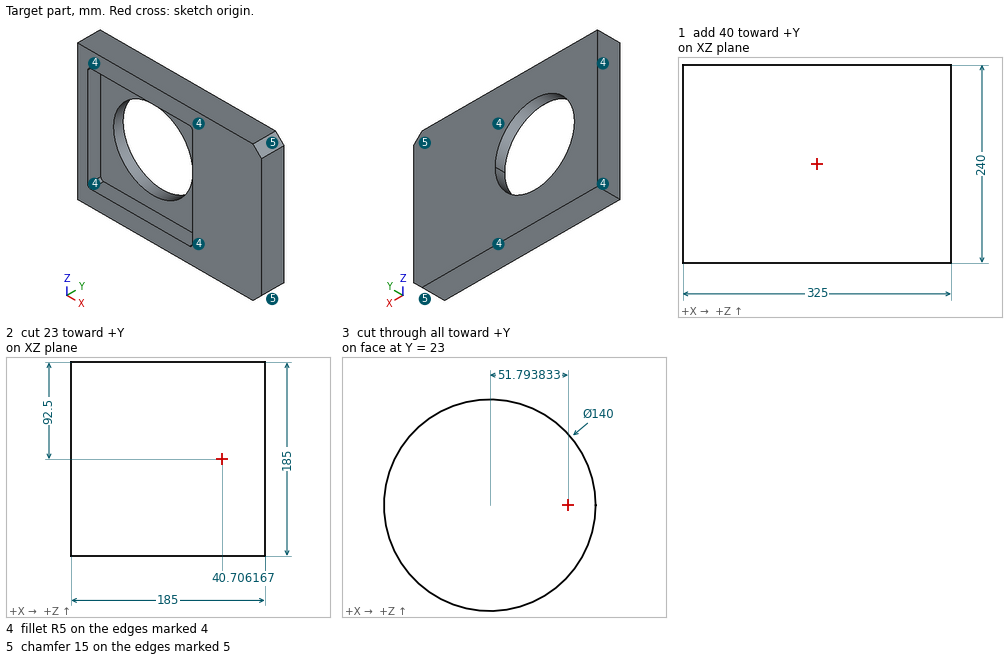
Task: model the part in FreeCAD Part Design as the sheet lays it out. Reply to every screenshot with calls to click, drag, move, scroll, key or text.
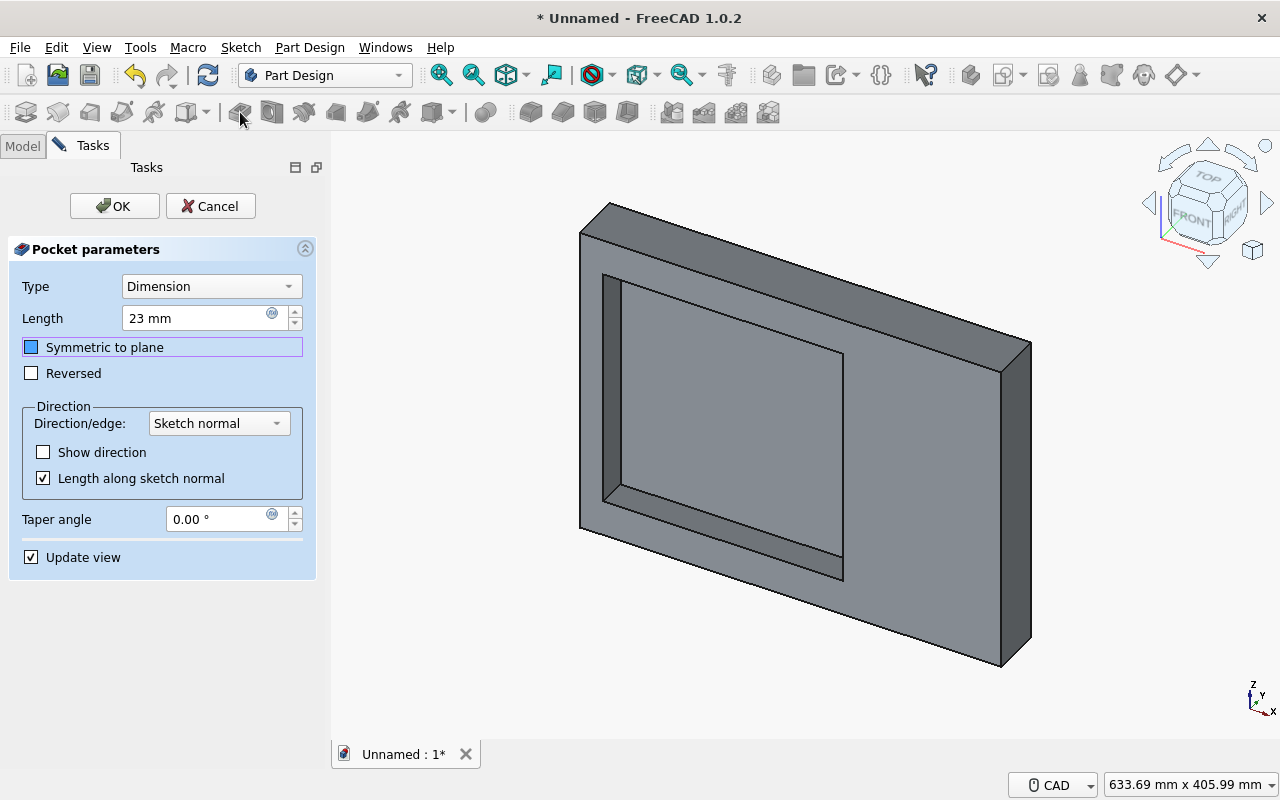
click(115, 206)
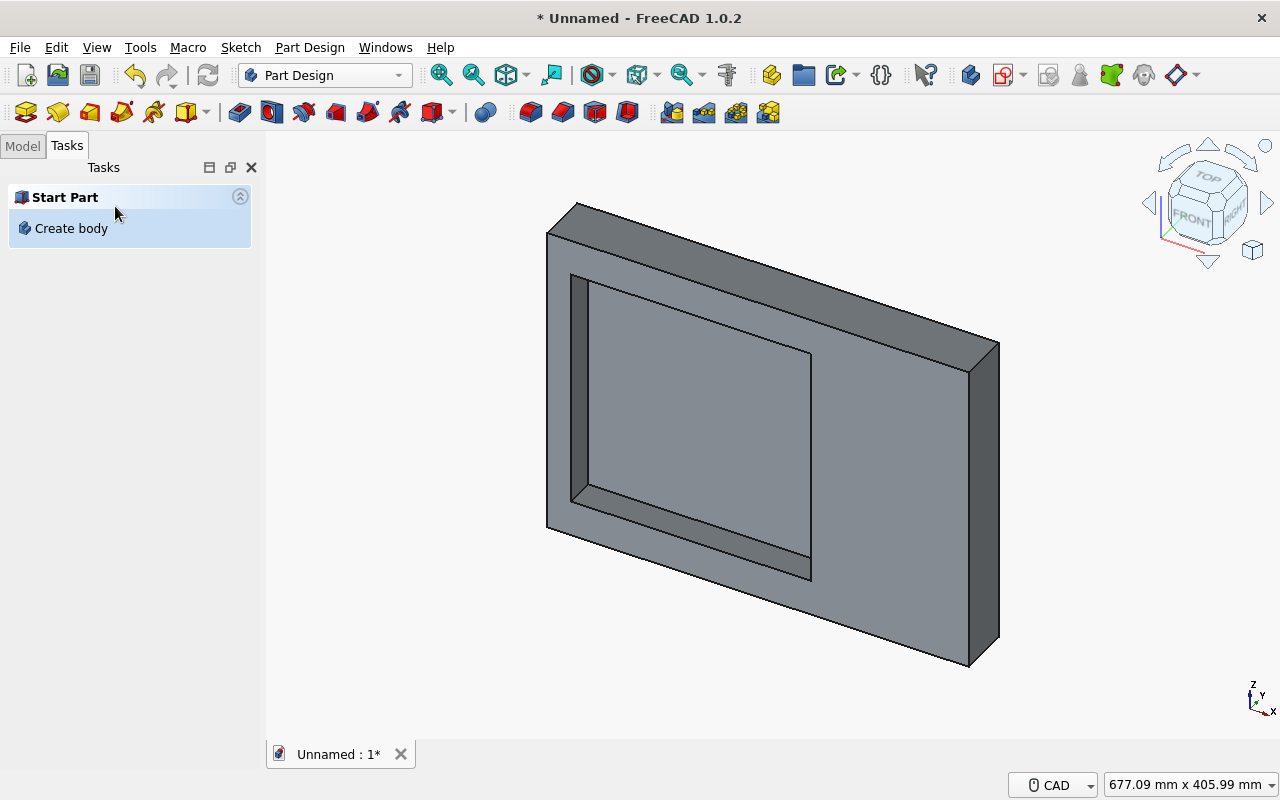
click(708, 410)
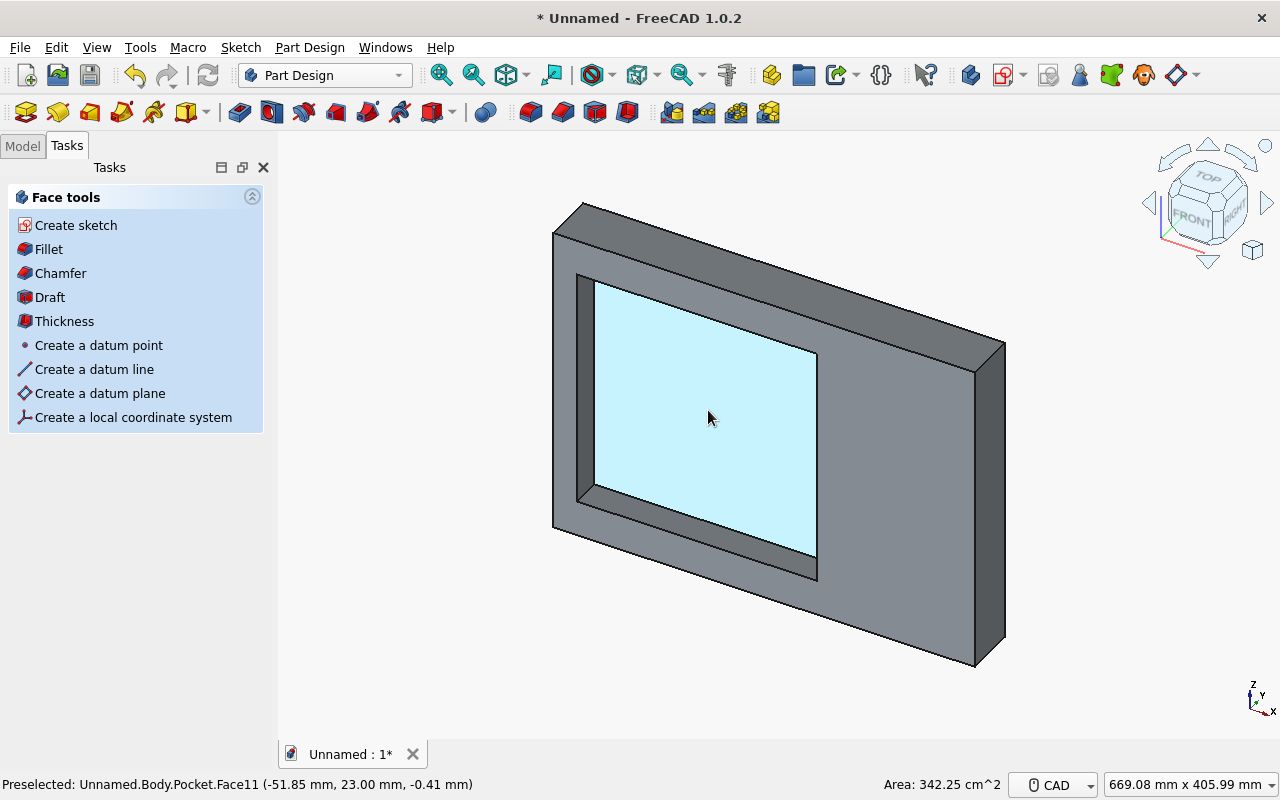
click(1004, 76)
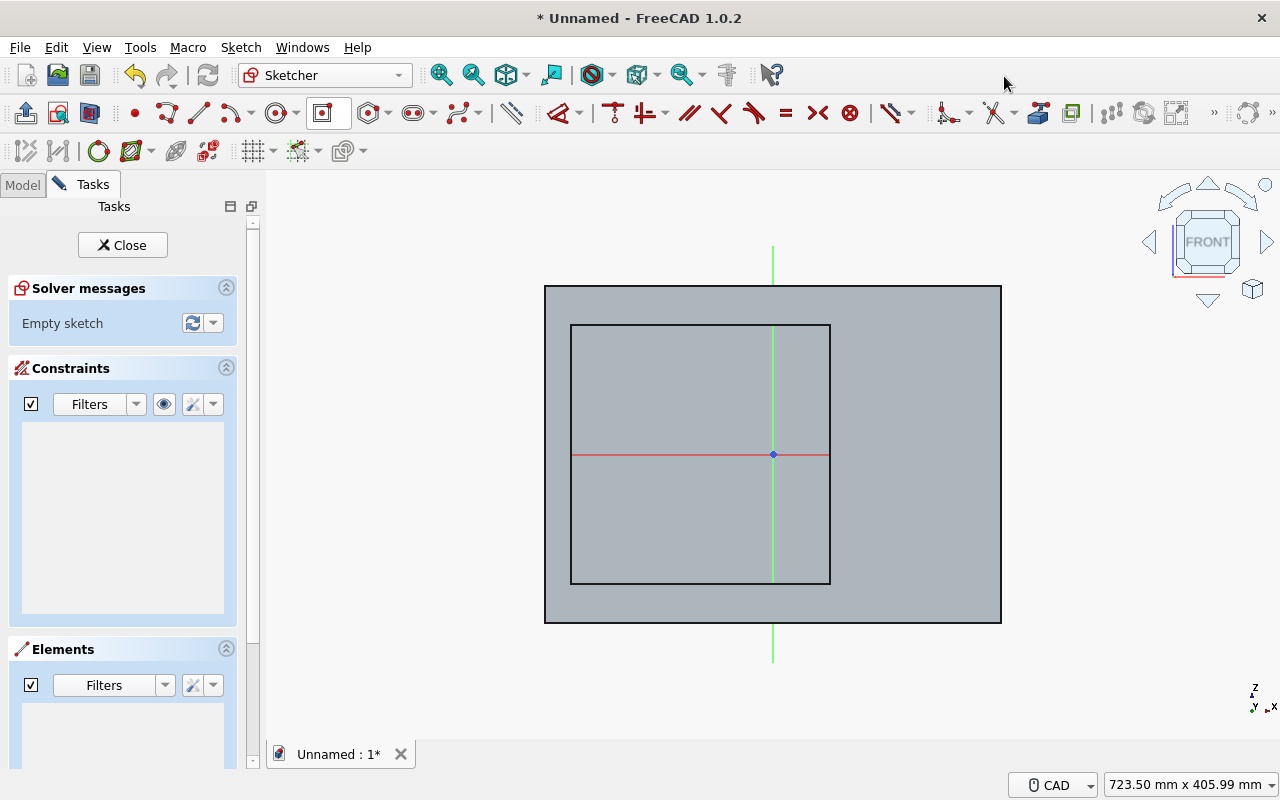
click(90, 114)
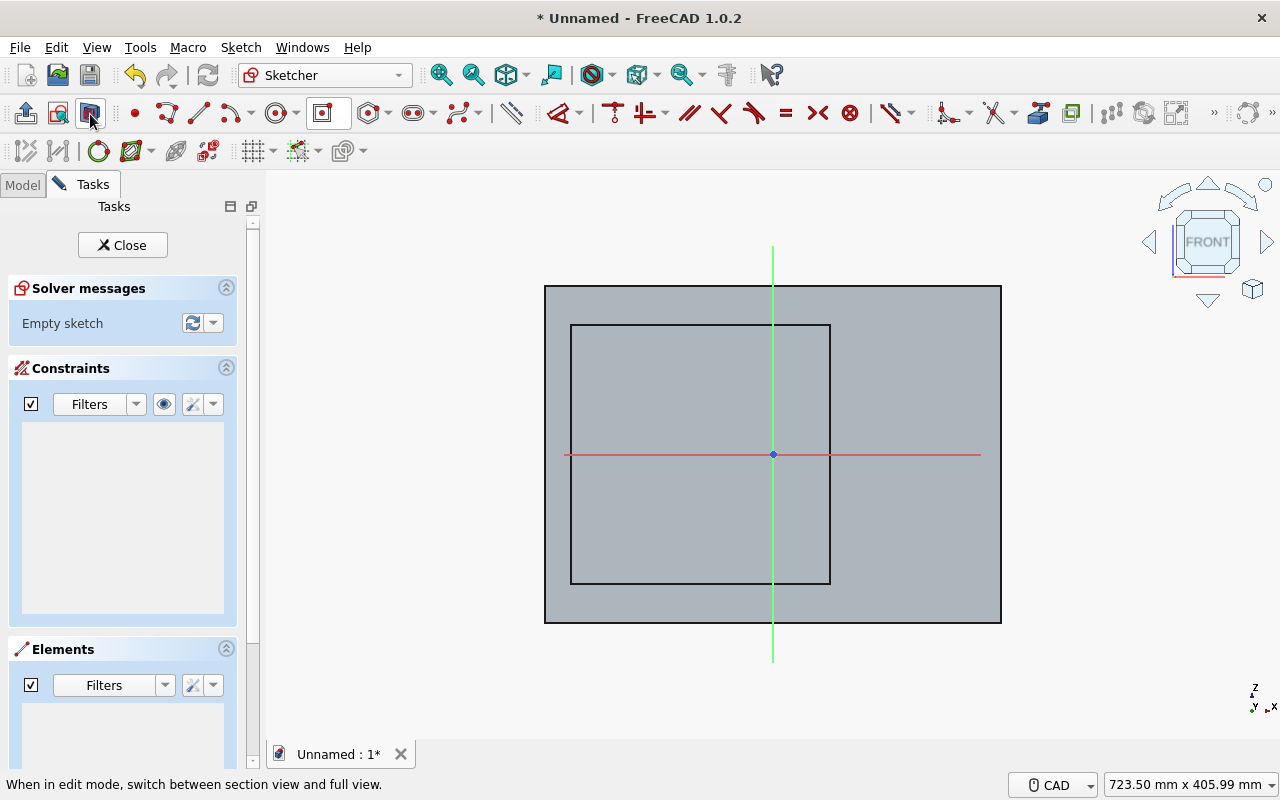
scroll(695, 455, up, 3)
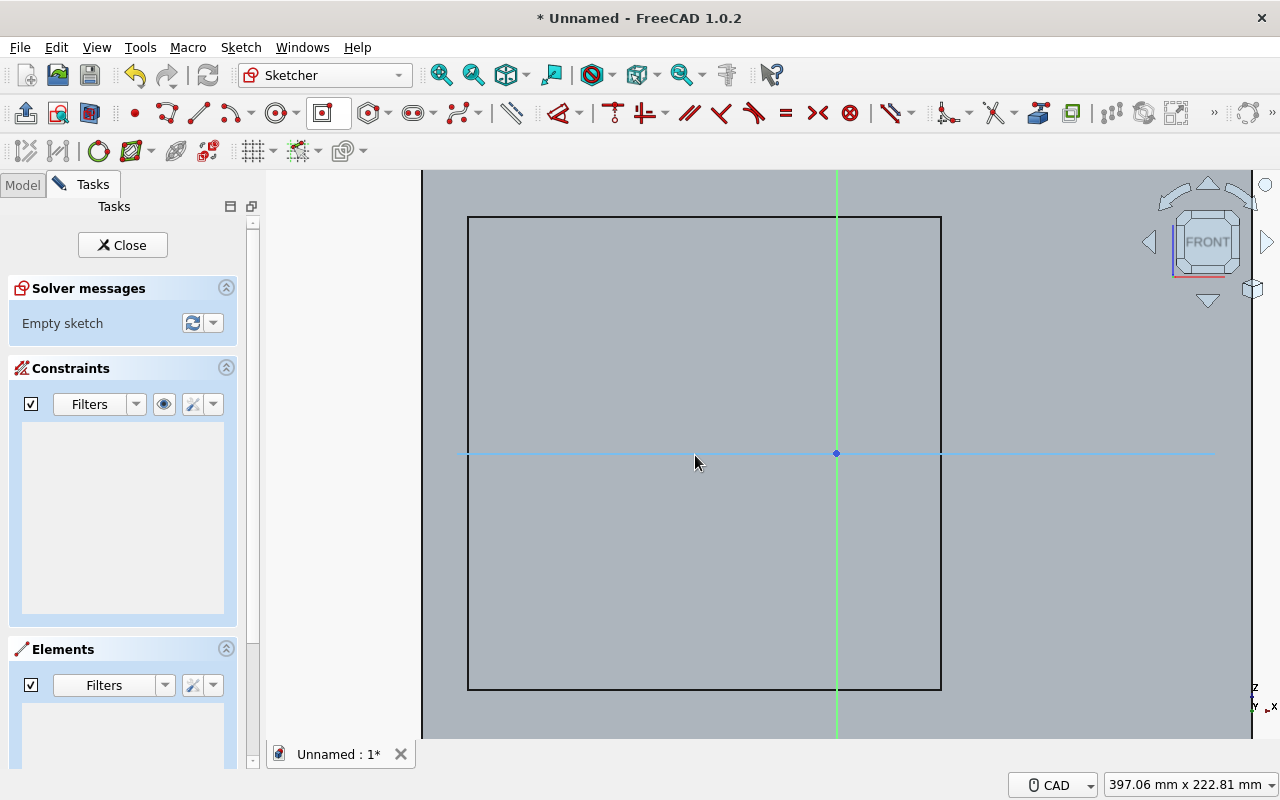
click(276, 114)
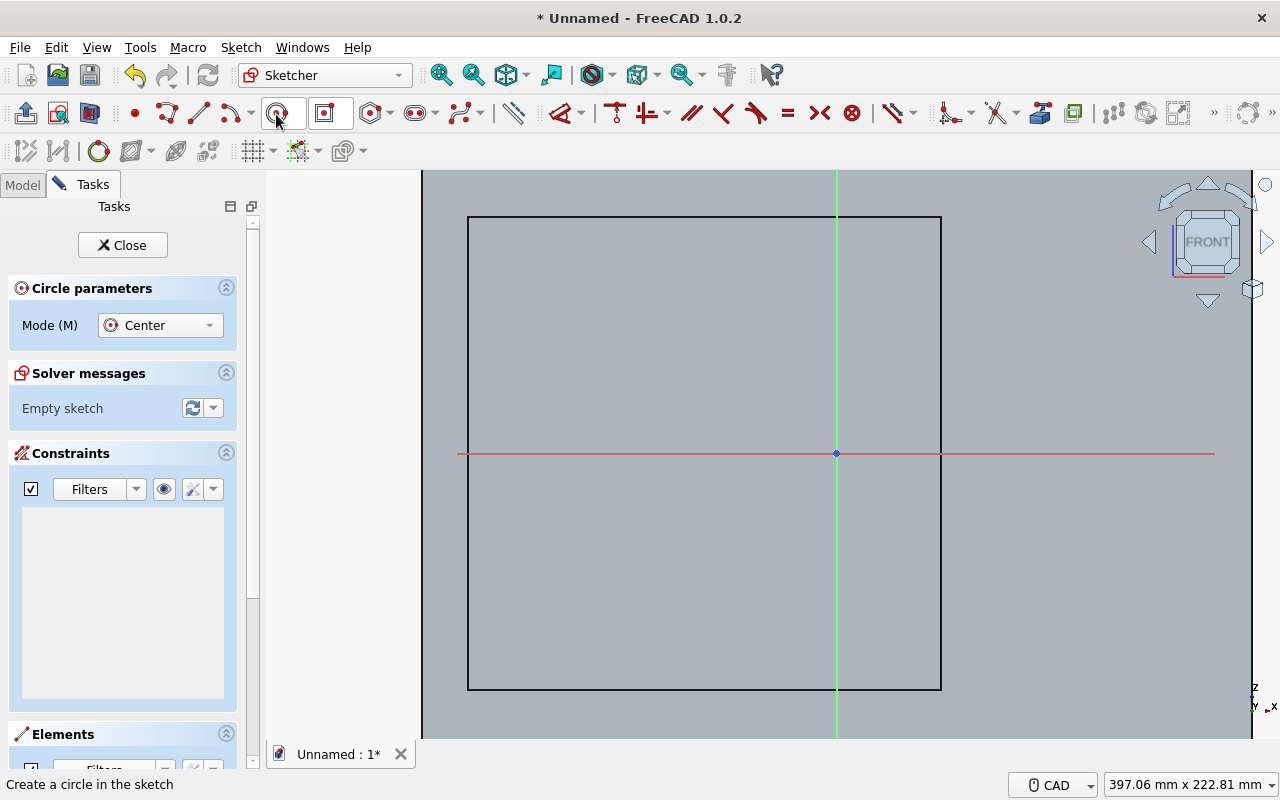
click(705, 454)
move(578, 327)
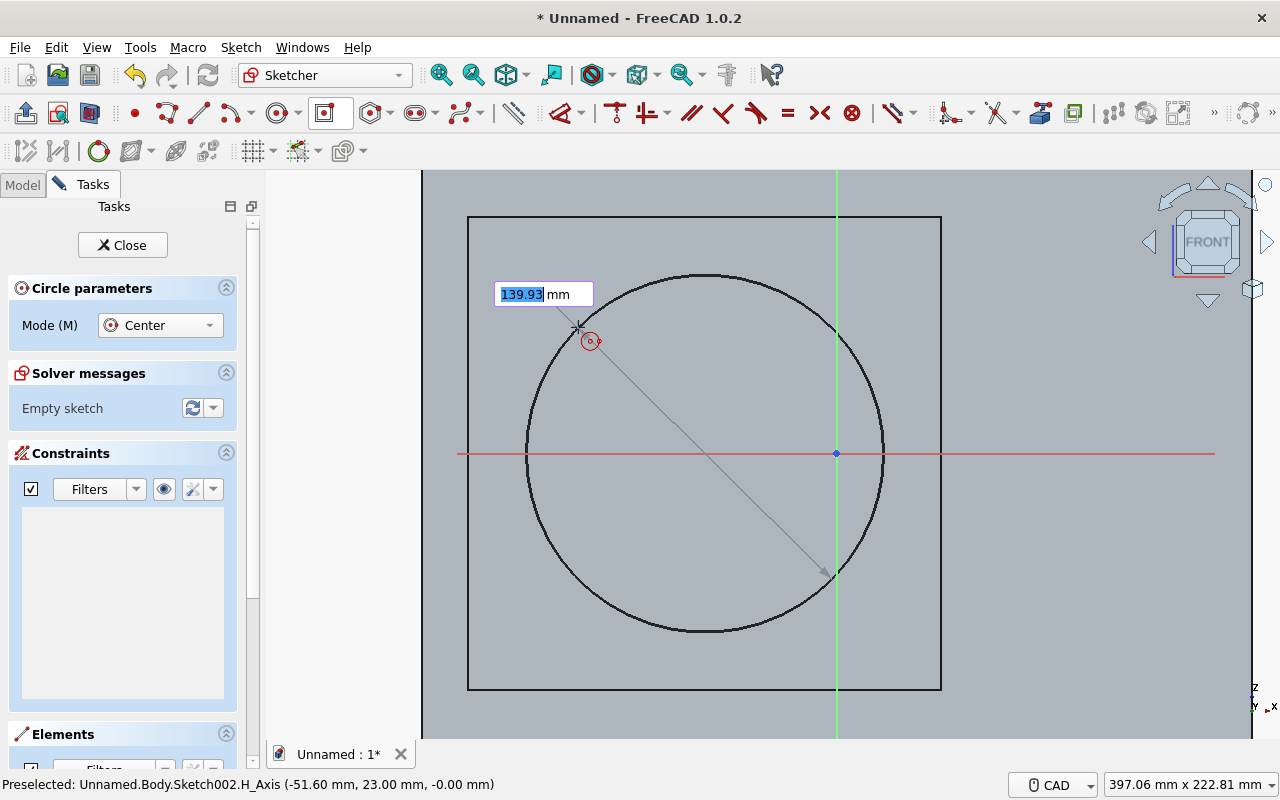
text(140)
key(Return)
key(Escape)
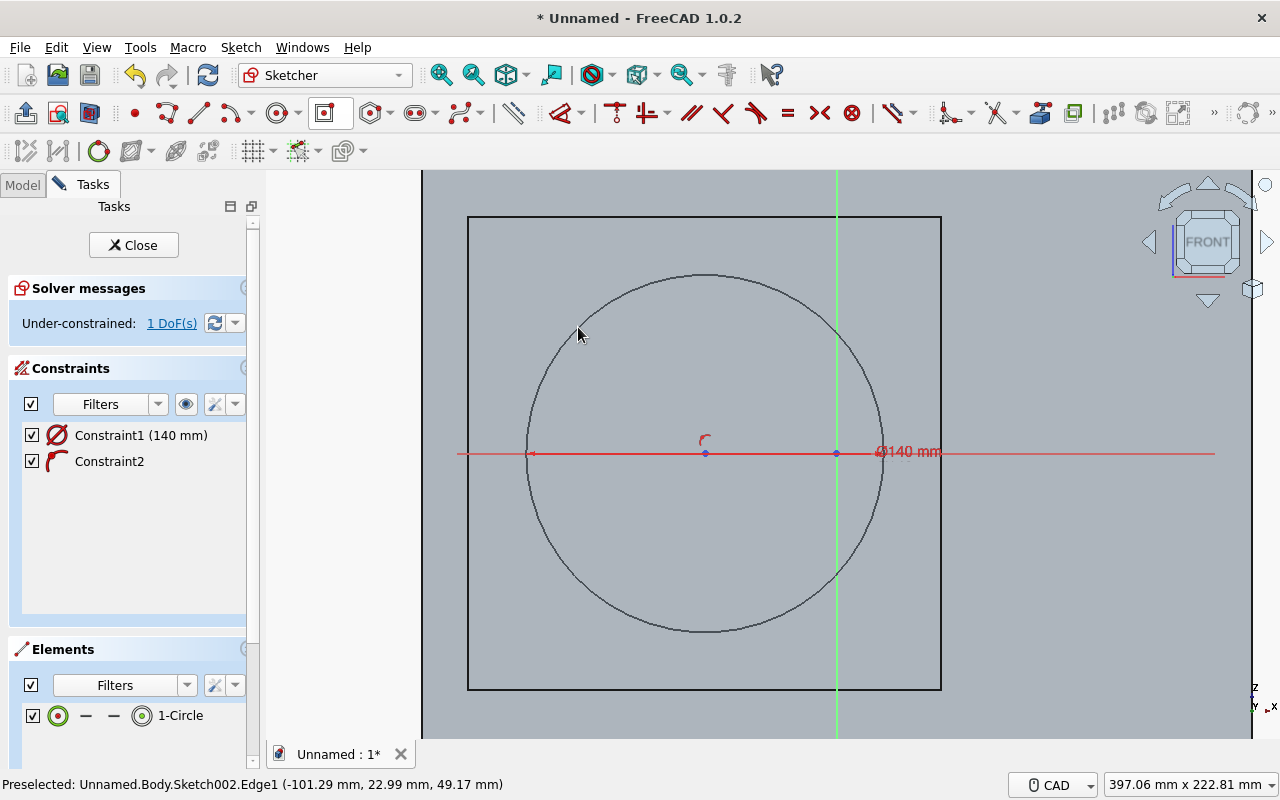
click(560, 114)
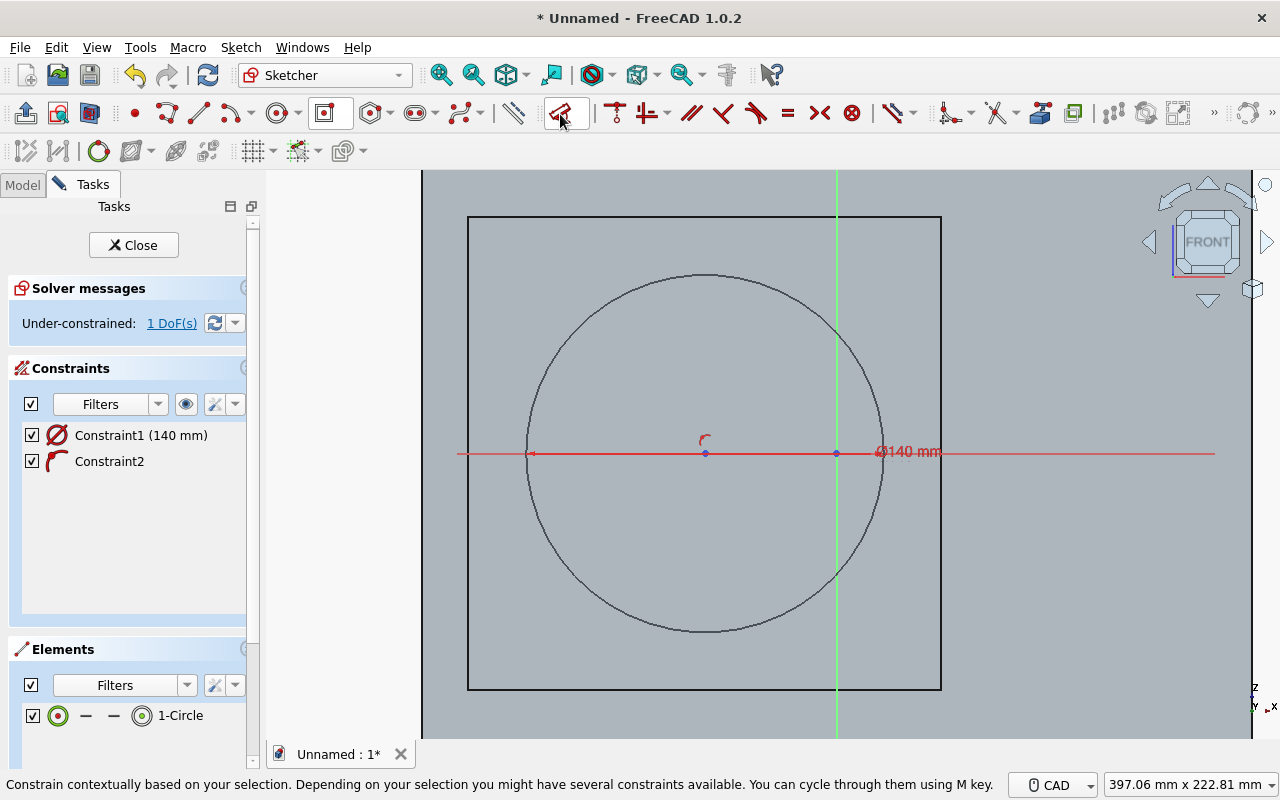
click(705, 454)
click(771, 488)